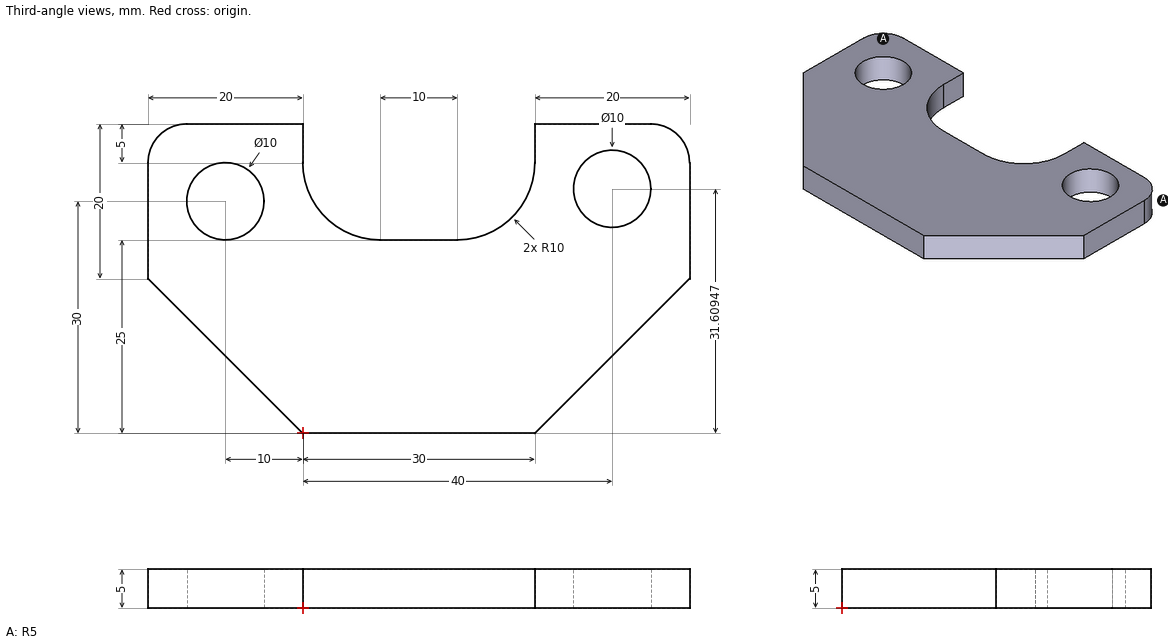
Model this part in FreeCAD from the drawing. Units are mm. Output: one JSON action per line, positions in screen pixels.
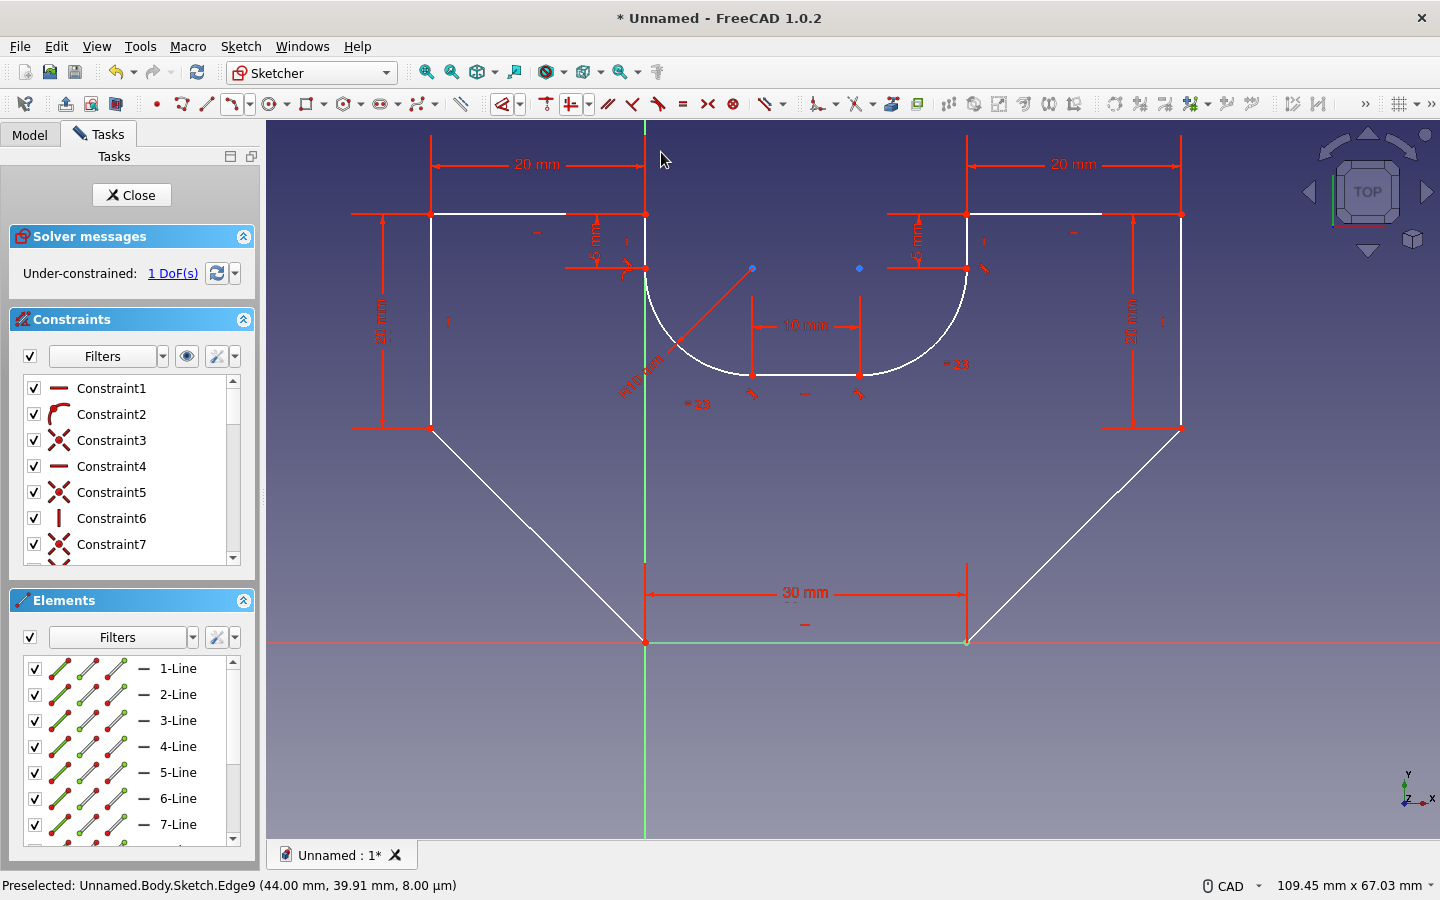
{"action": "left_click", "coordinate": [860, 375]}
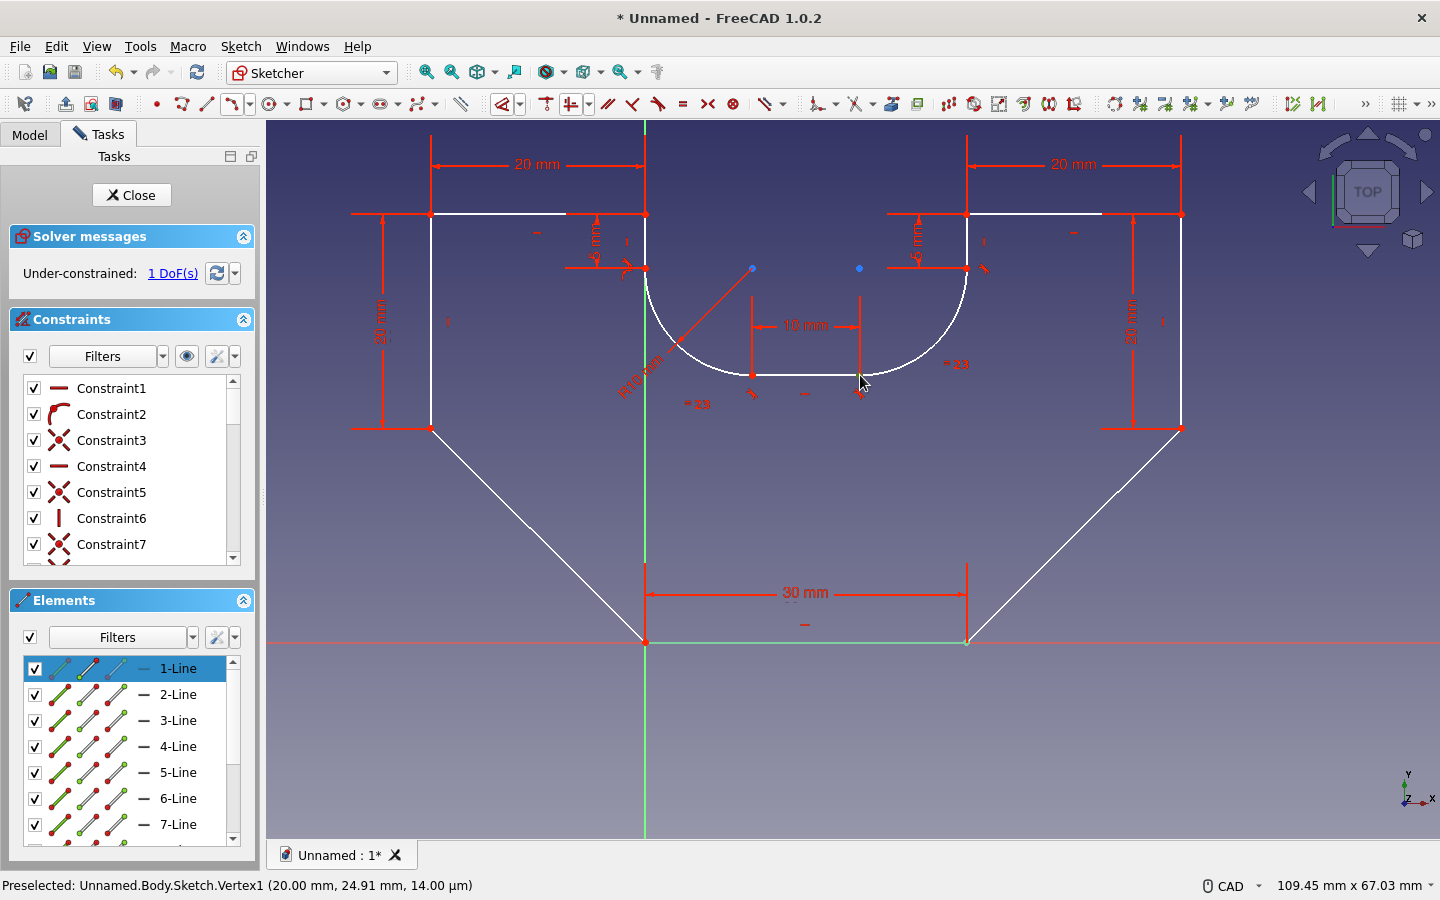
{"action": "left_click", "coordinate": [520, 104]}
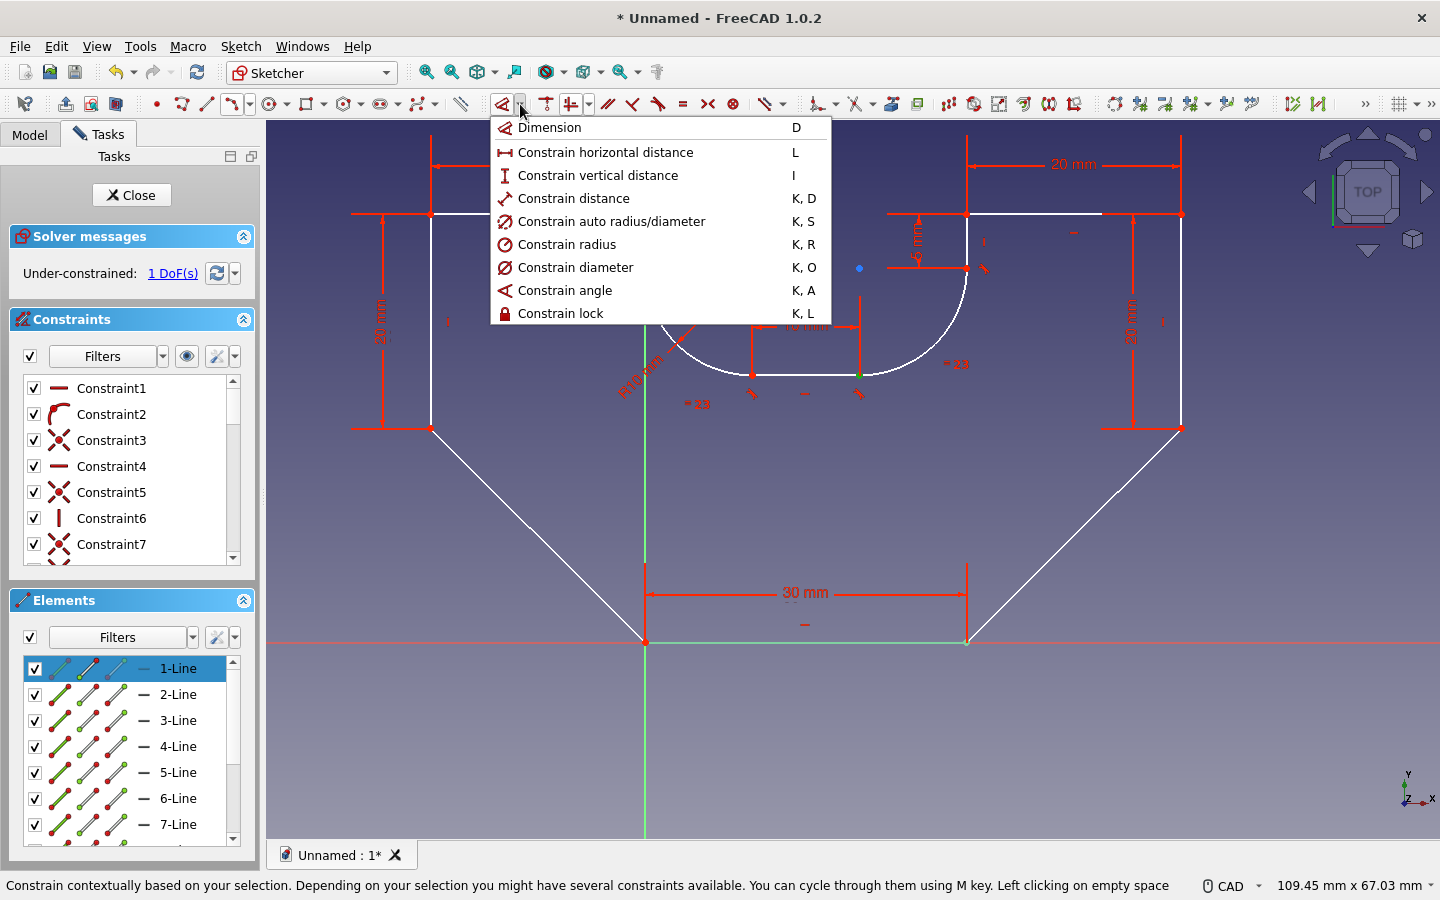
{"action": "left_click", "coordinate": [661, 176]}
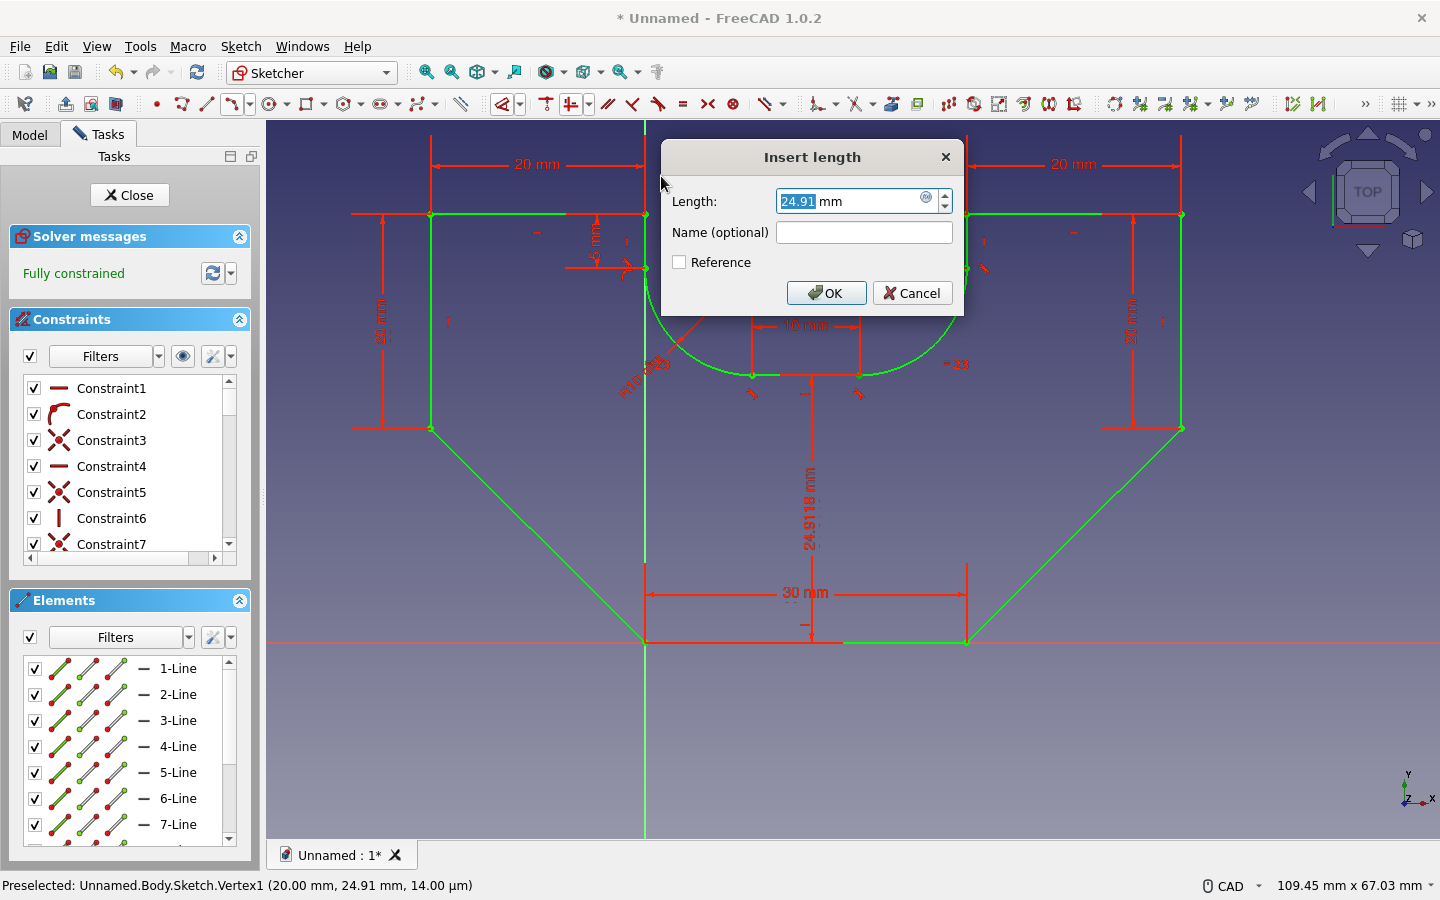
{"action": "type", "text": "25"}
{"action": "key", "text": "Return"}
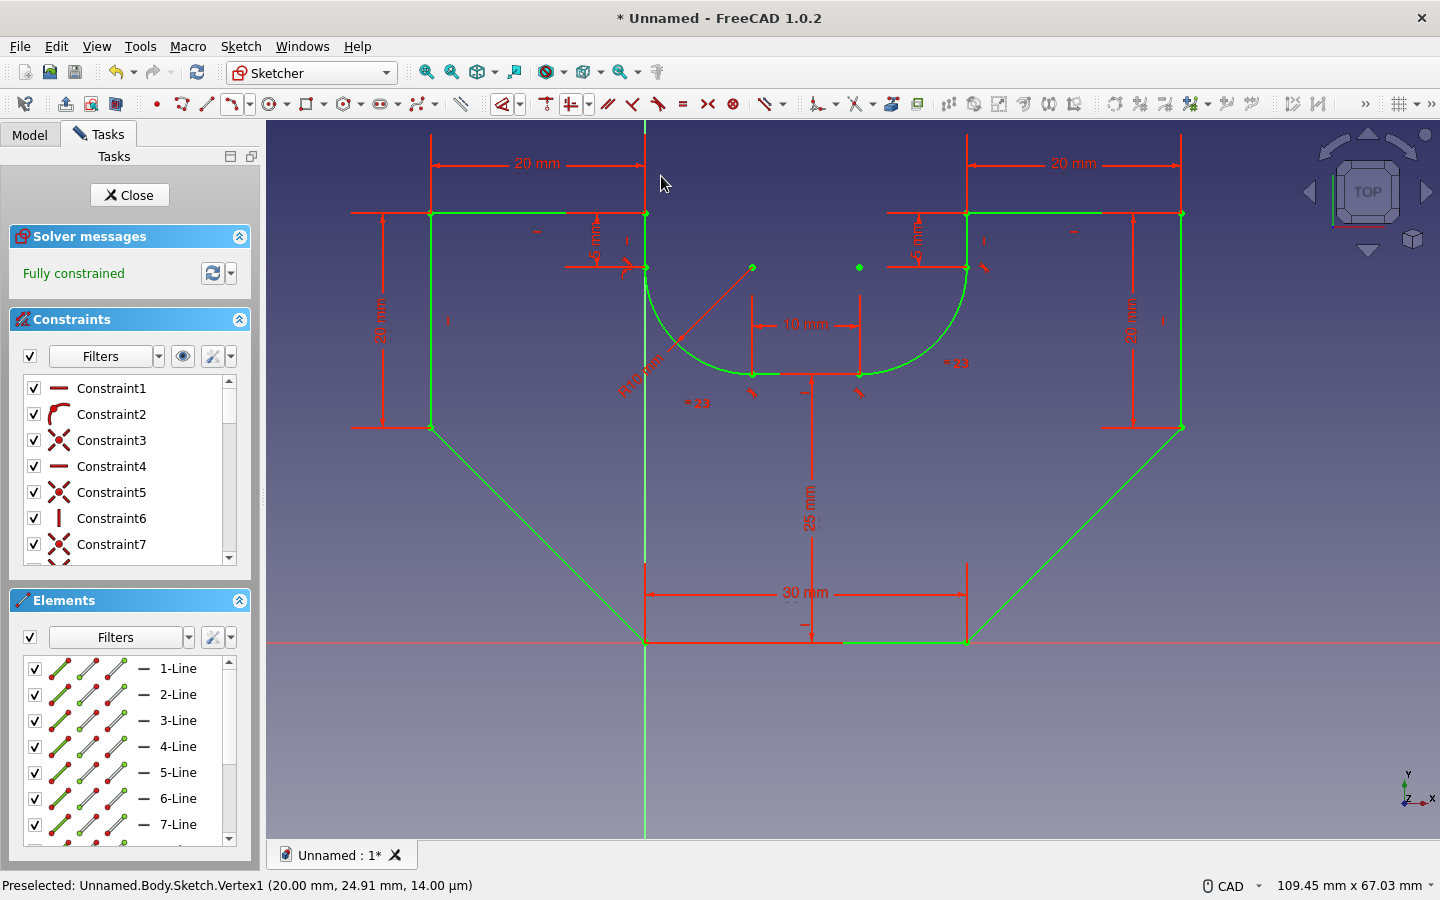
{"action": "left_click", "coordinate": [130, 195]}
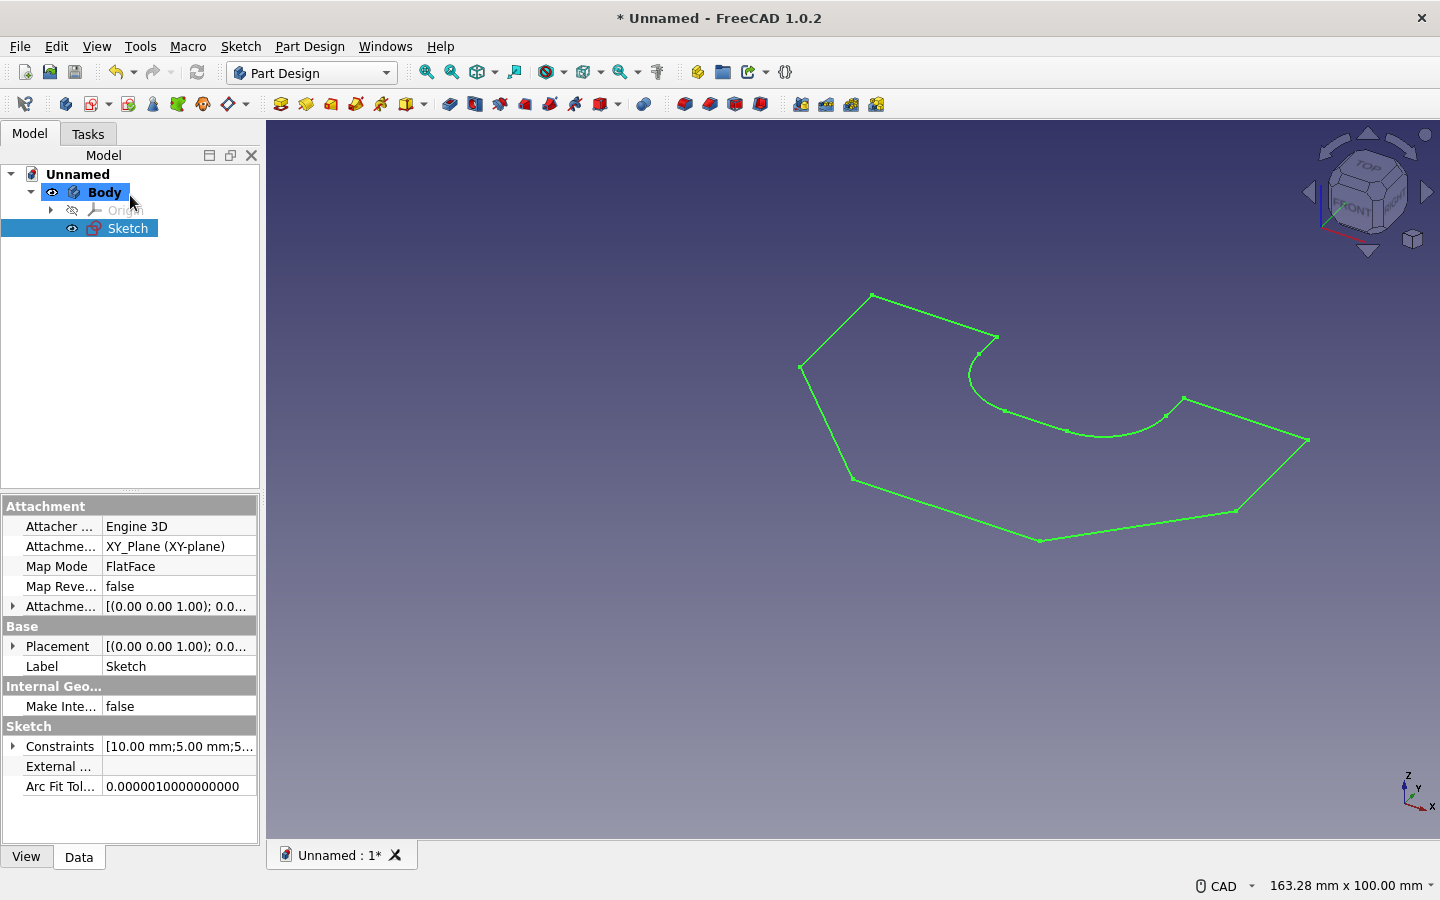
{"action": "left_click", "coordinate": [281, 104]}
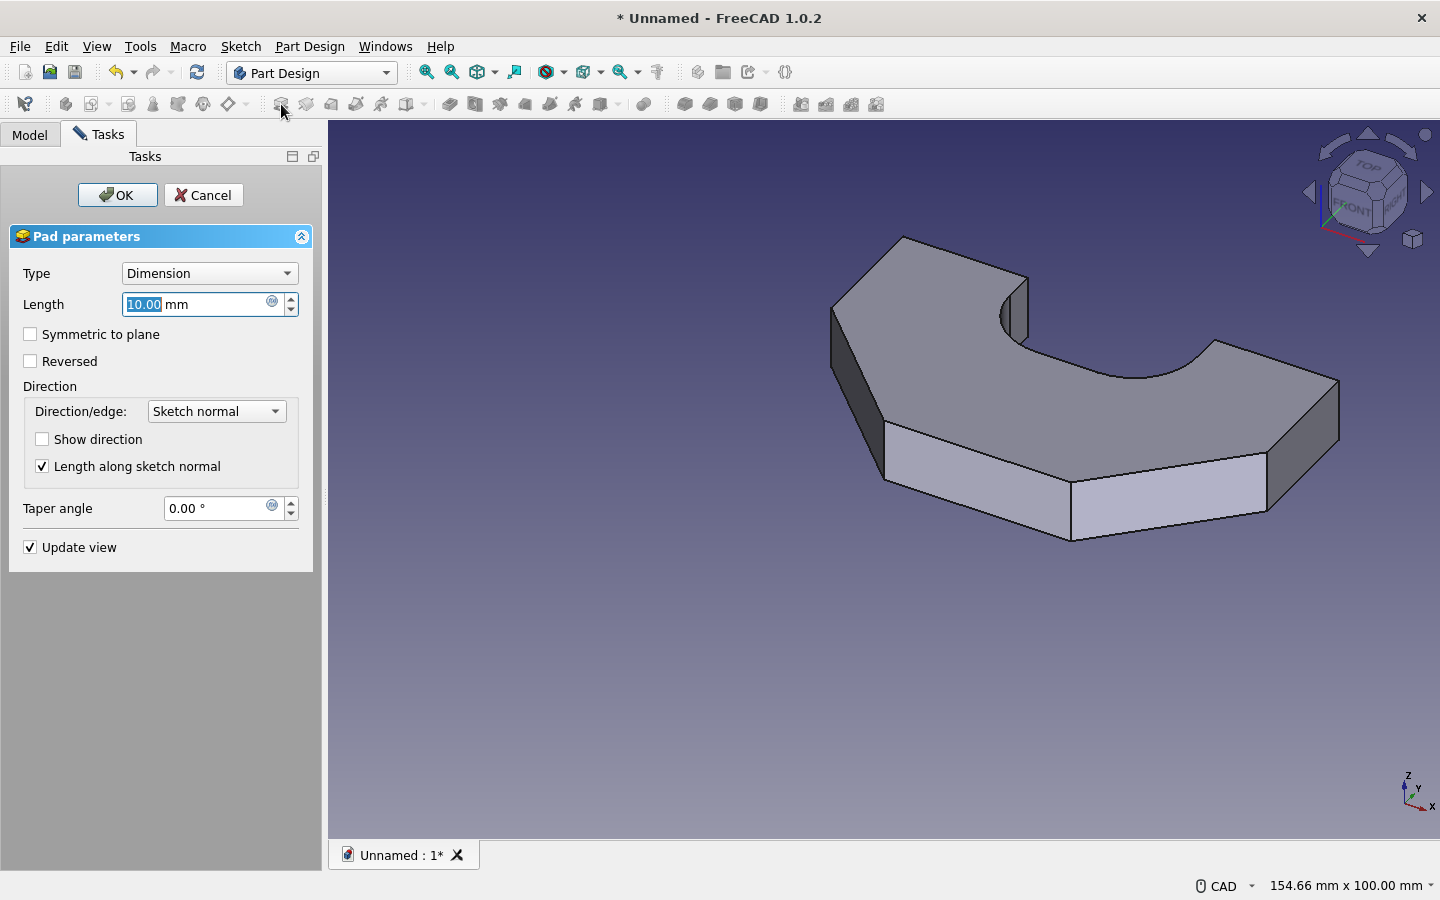
{"action": "type", "text": "5"}
{"action": "key", "text": "Tab"}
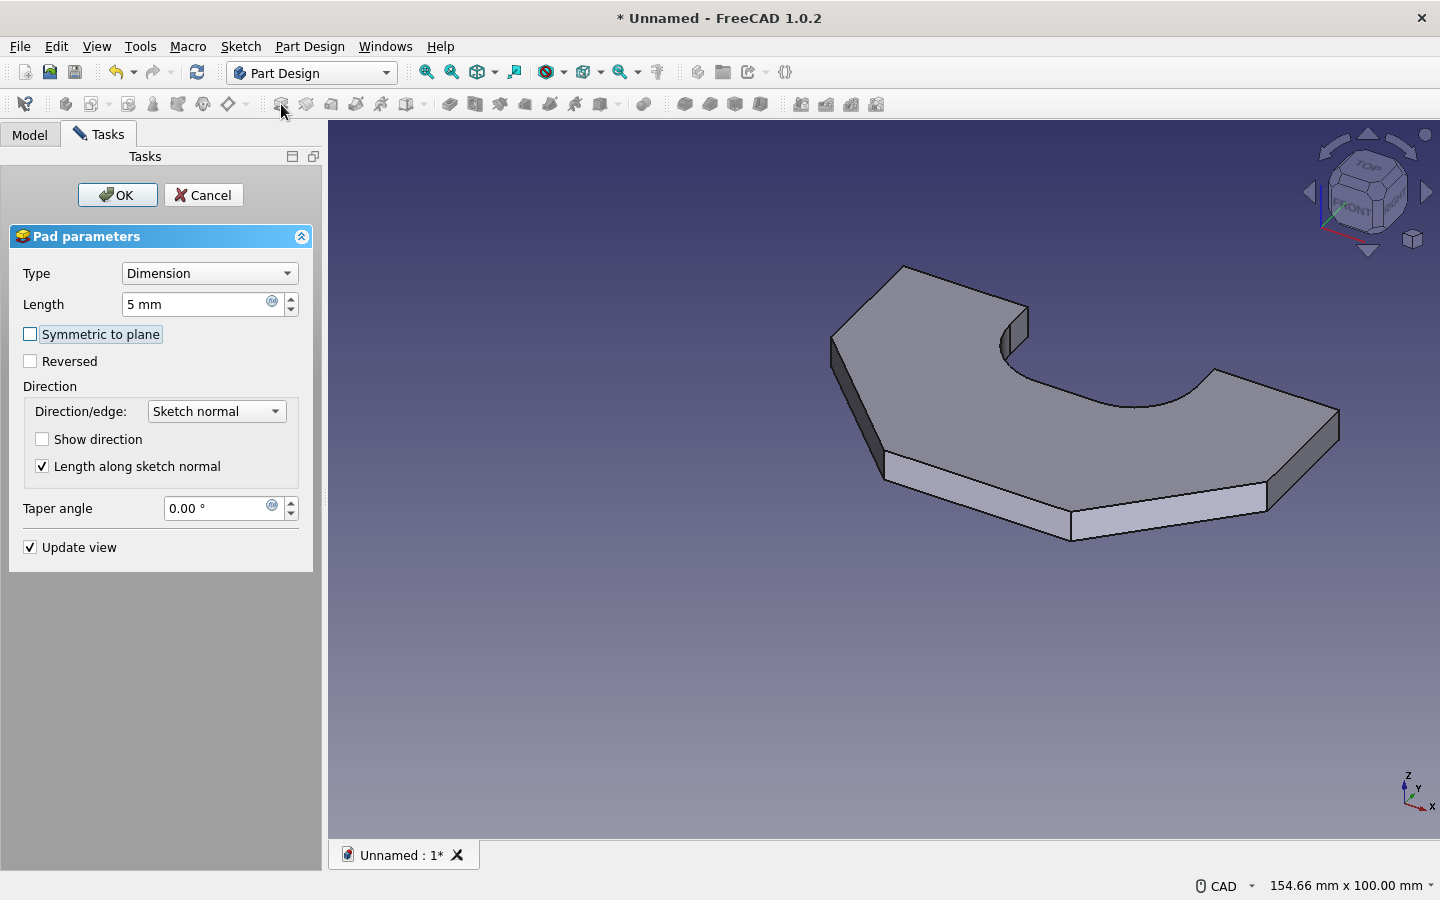
{"action": "left_click", "coordinate": [118, 195]}